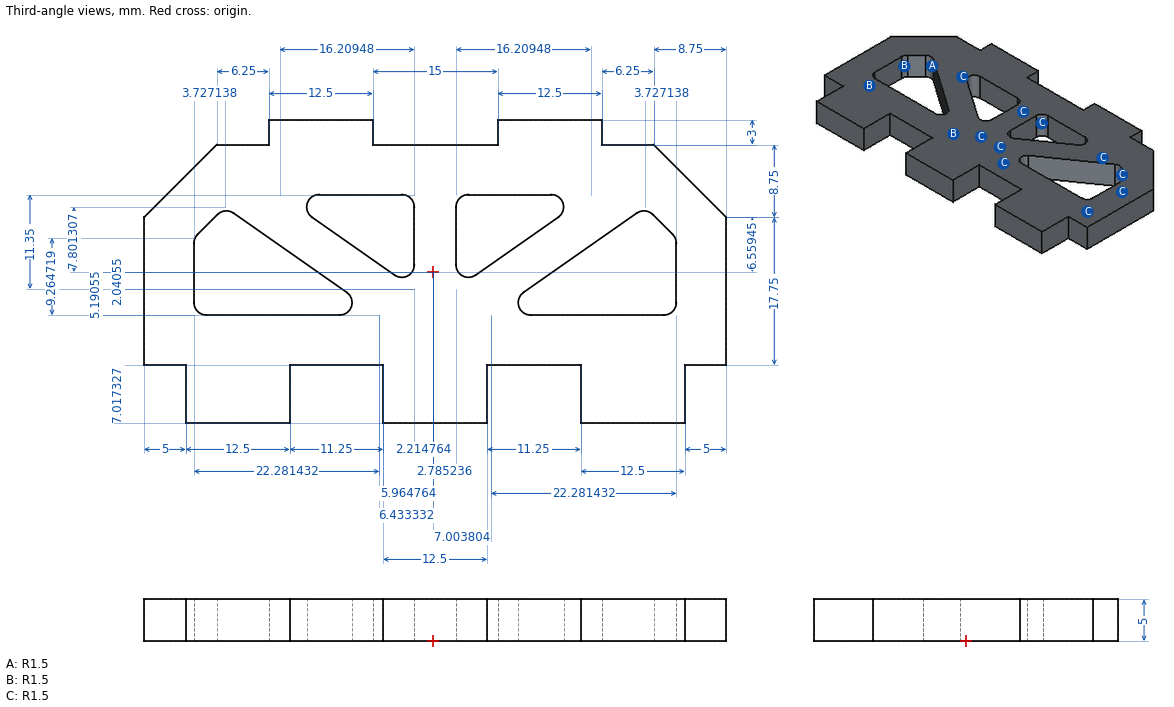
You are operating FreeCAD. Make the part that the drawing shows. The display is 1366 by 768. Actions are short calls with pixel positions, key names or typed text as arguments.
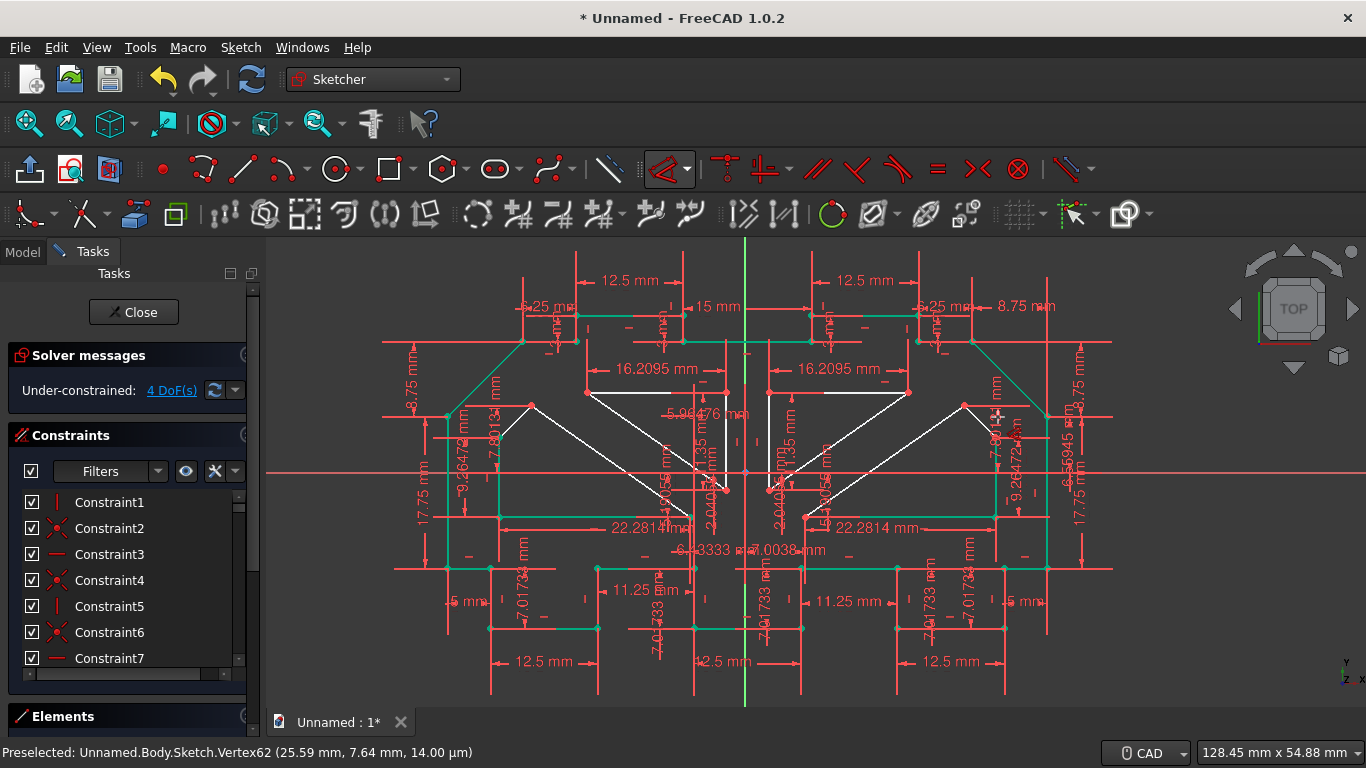
scroll(726, 490, up, 4)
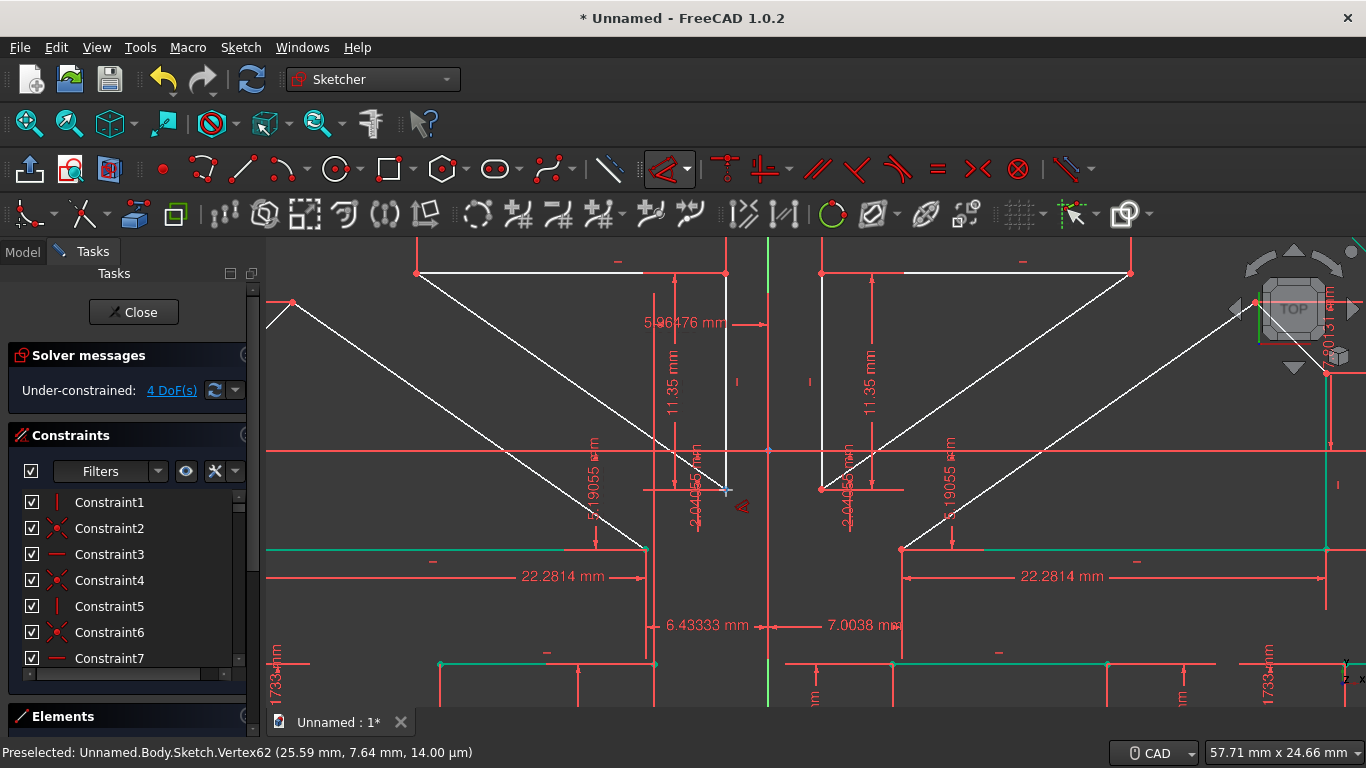
click(726, 490)
click(747, 524)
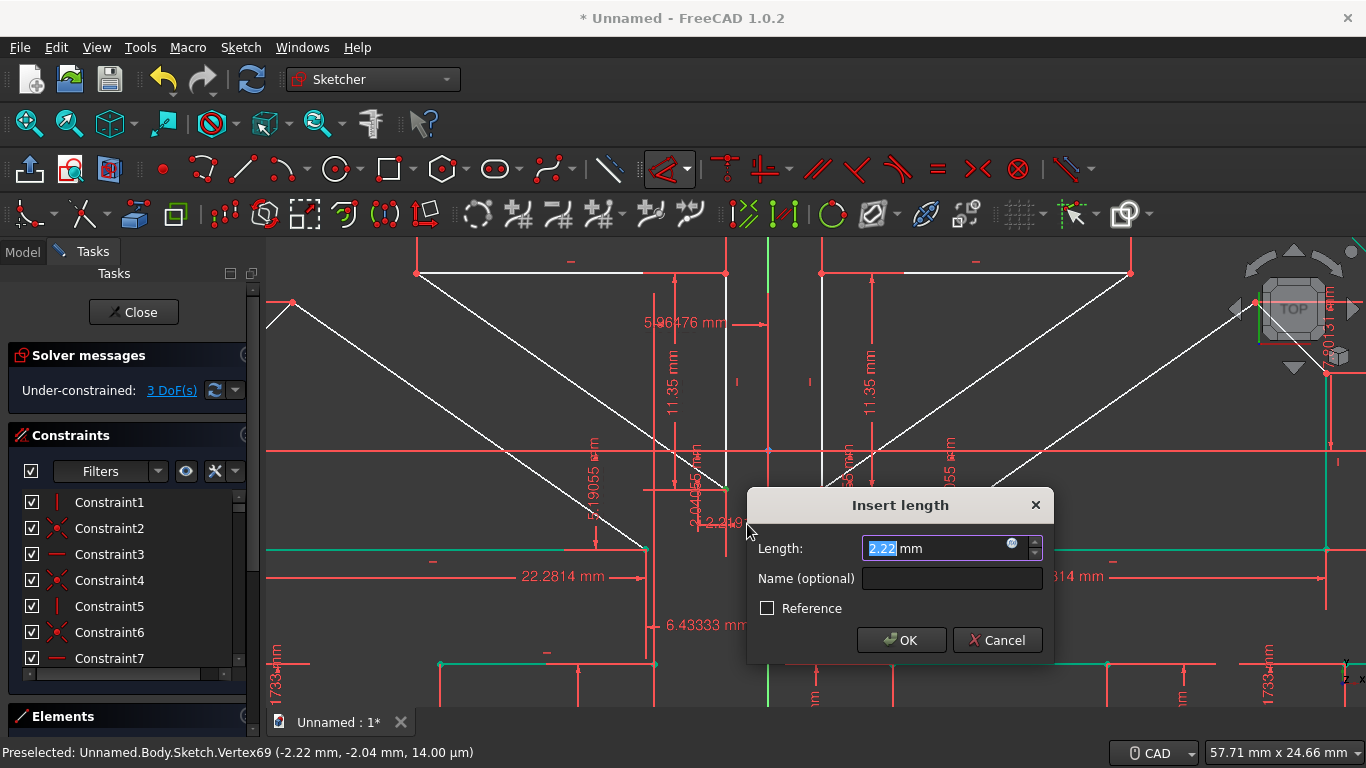
text(2.214764)
key(Return)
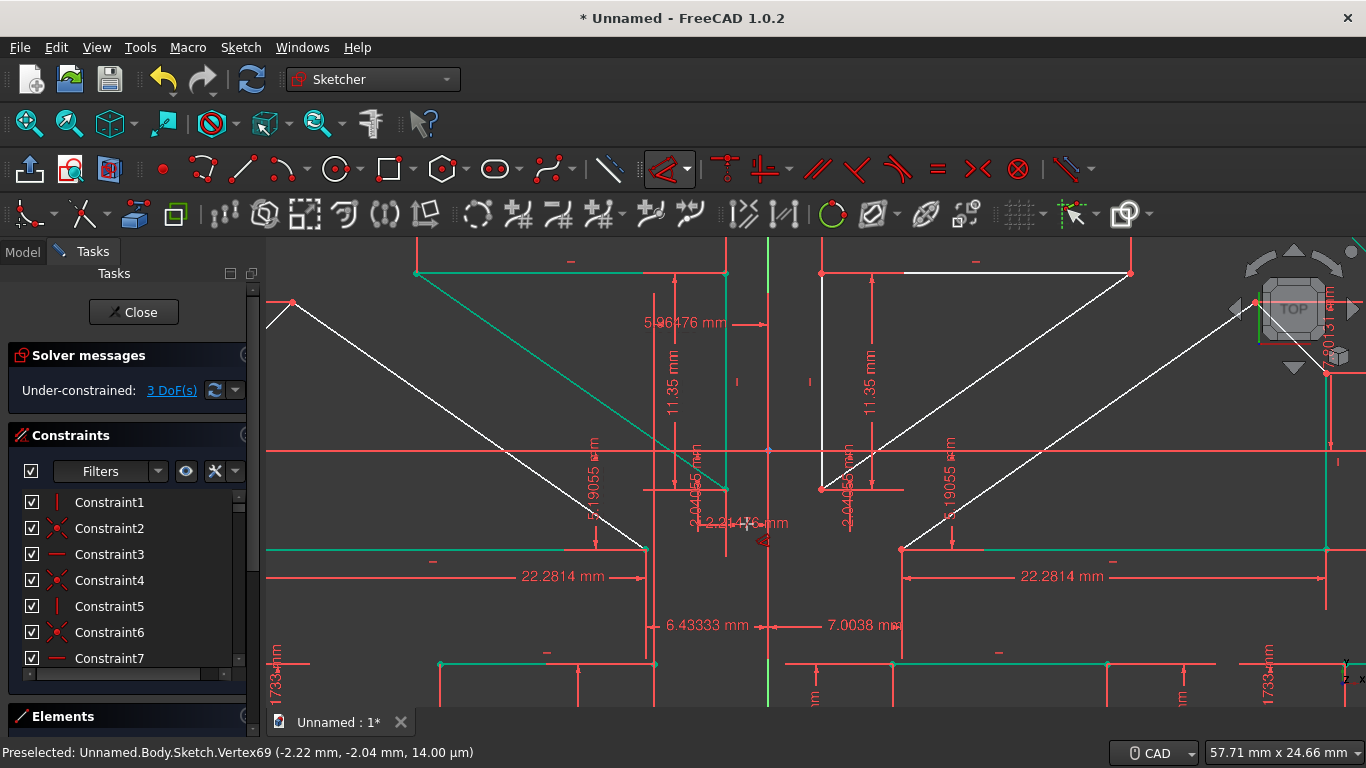
click(822, 490)
click(795, 417)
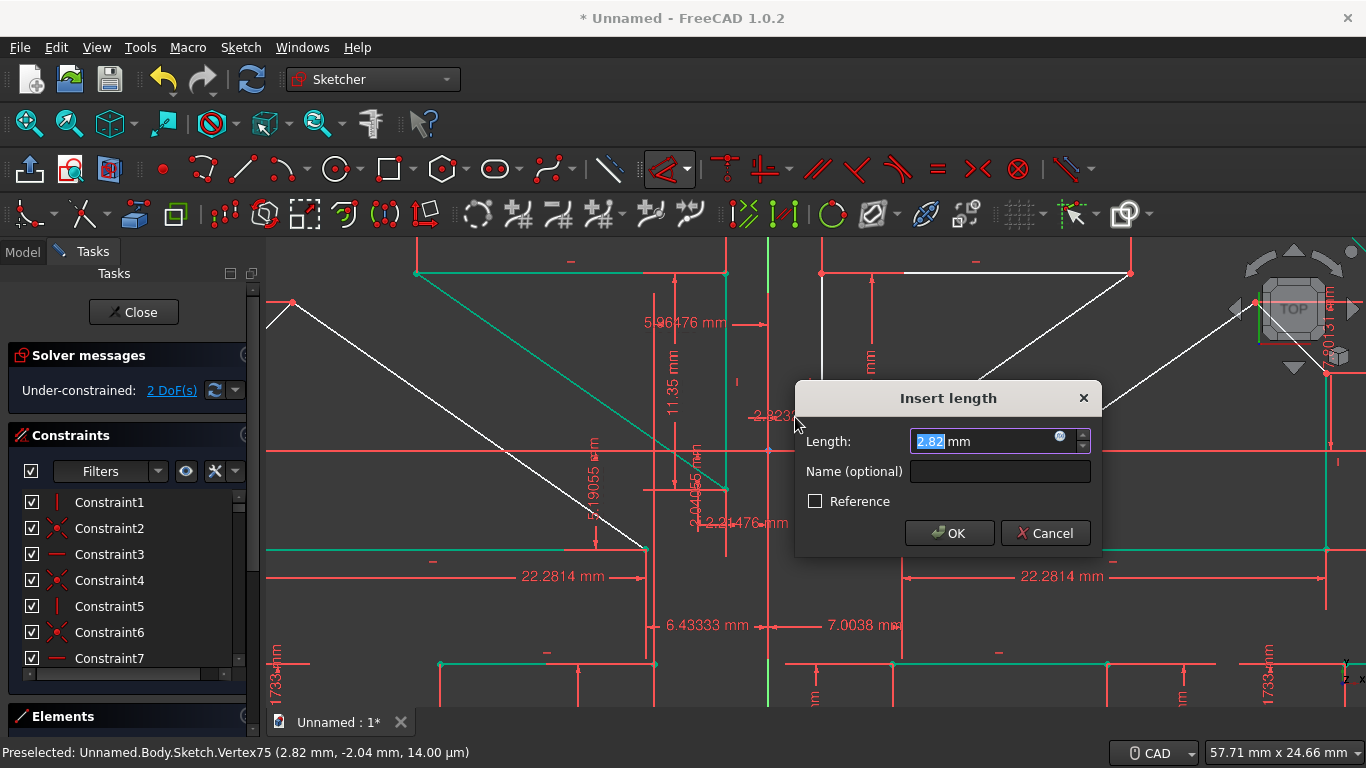
text(2.785236)
key(Return)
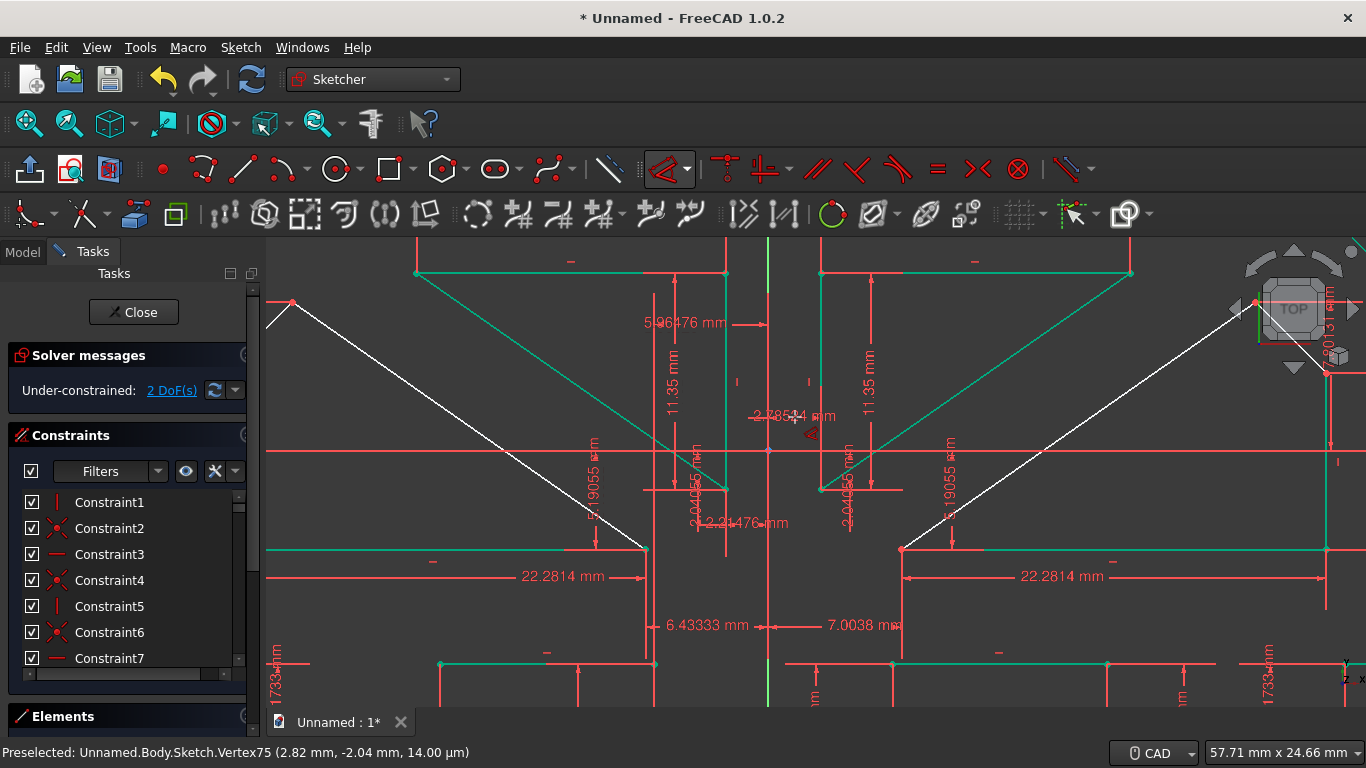
scroll(726, 490, down, 4)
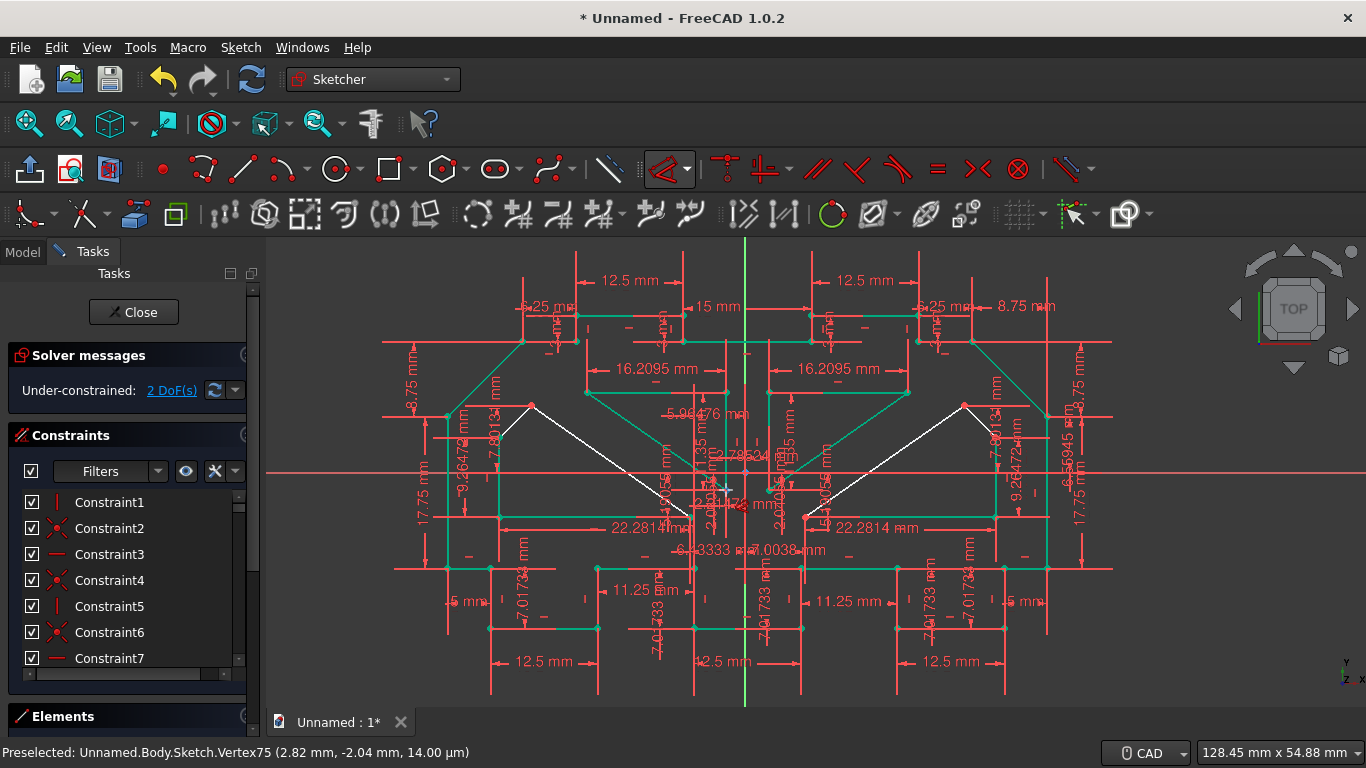
scroll(509, 428, up, 2)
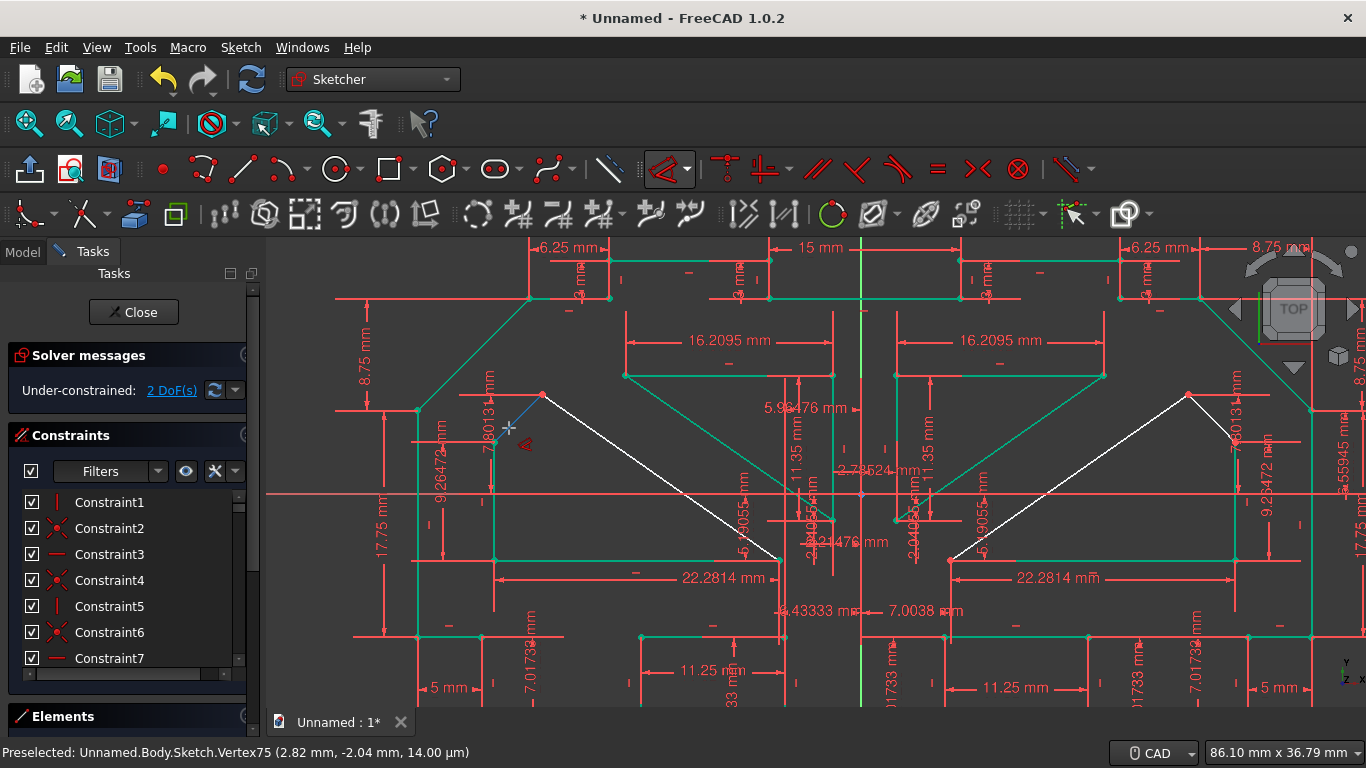
click(509, 428)
click(518, 361)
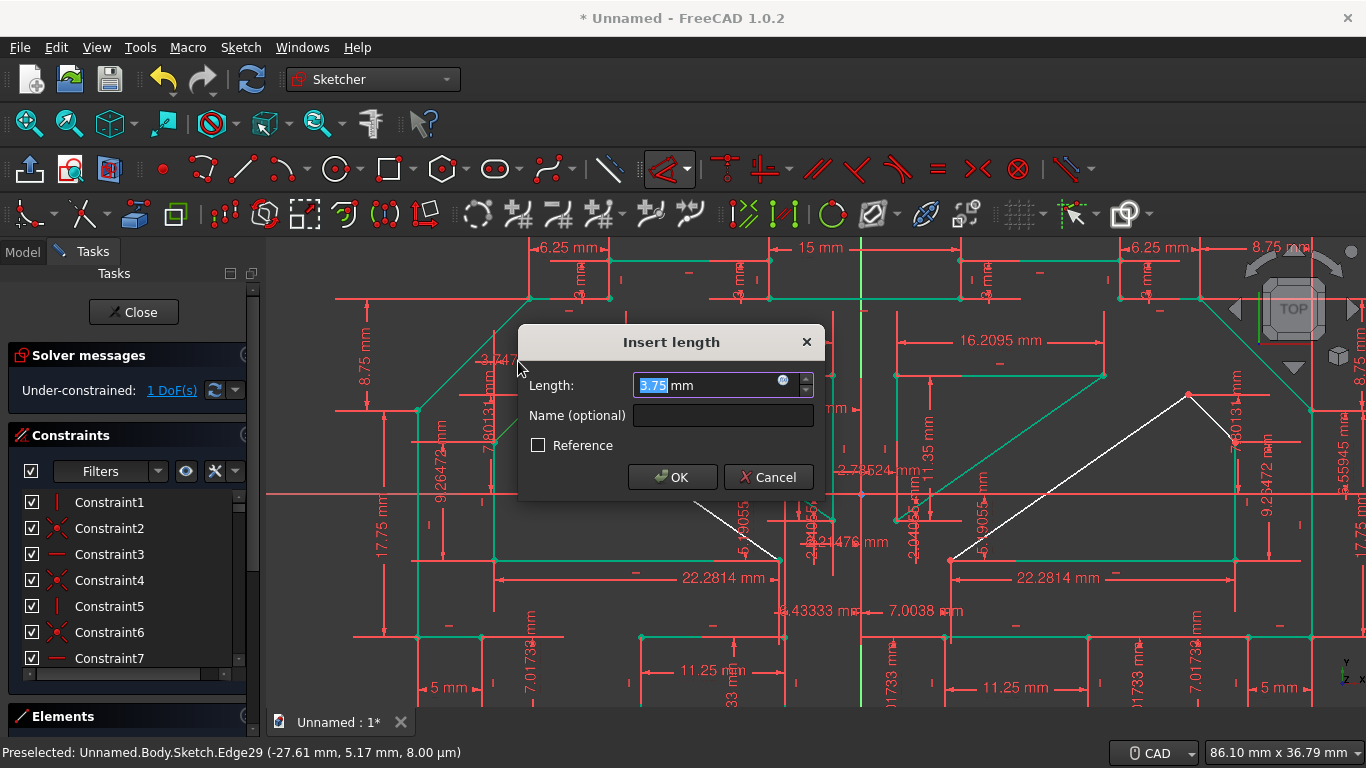
text(3.727138)
key(Return)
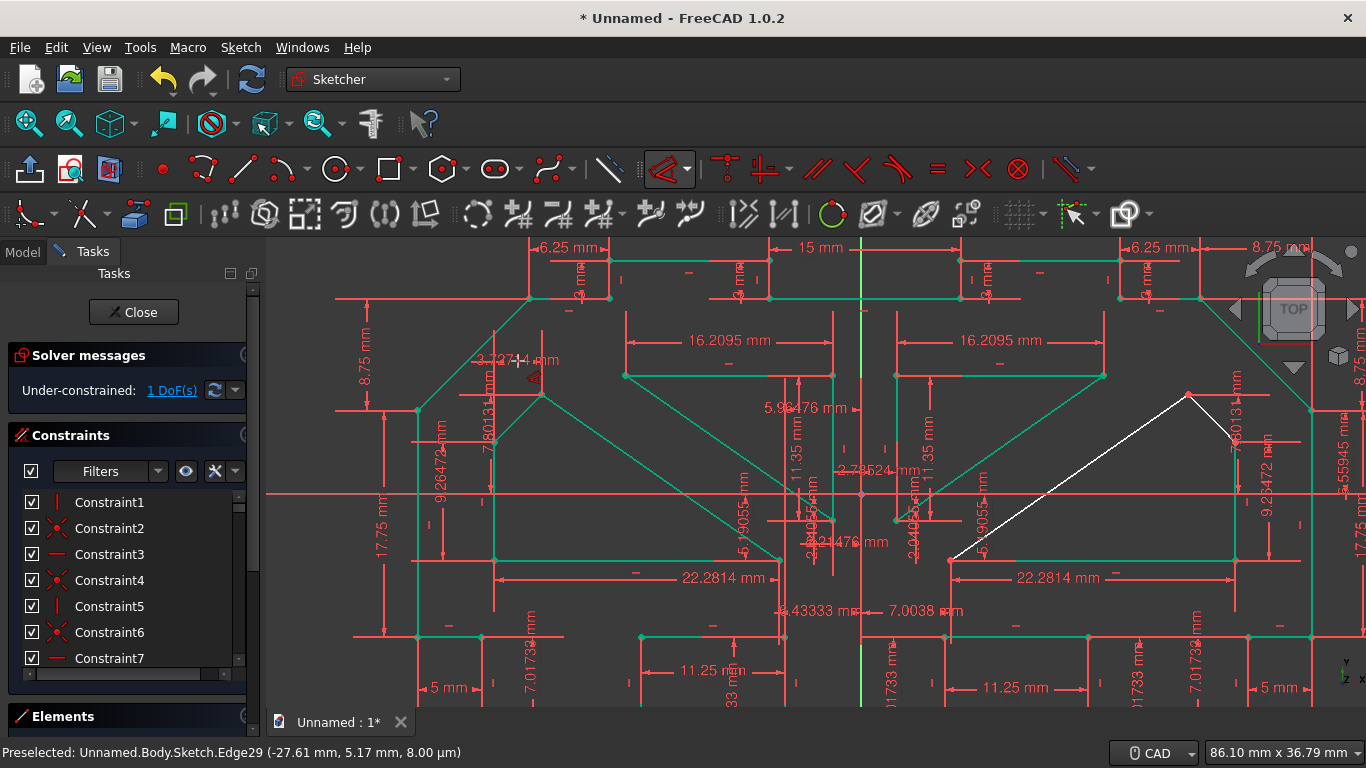
click(1198, 404)
click(1195, 361)